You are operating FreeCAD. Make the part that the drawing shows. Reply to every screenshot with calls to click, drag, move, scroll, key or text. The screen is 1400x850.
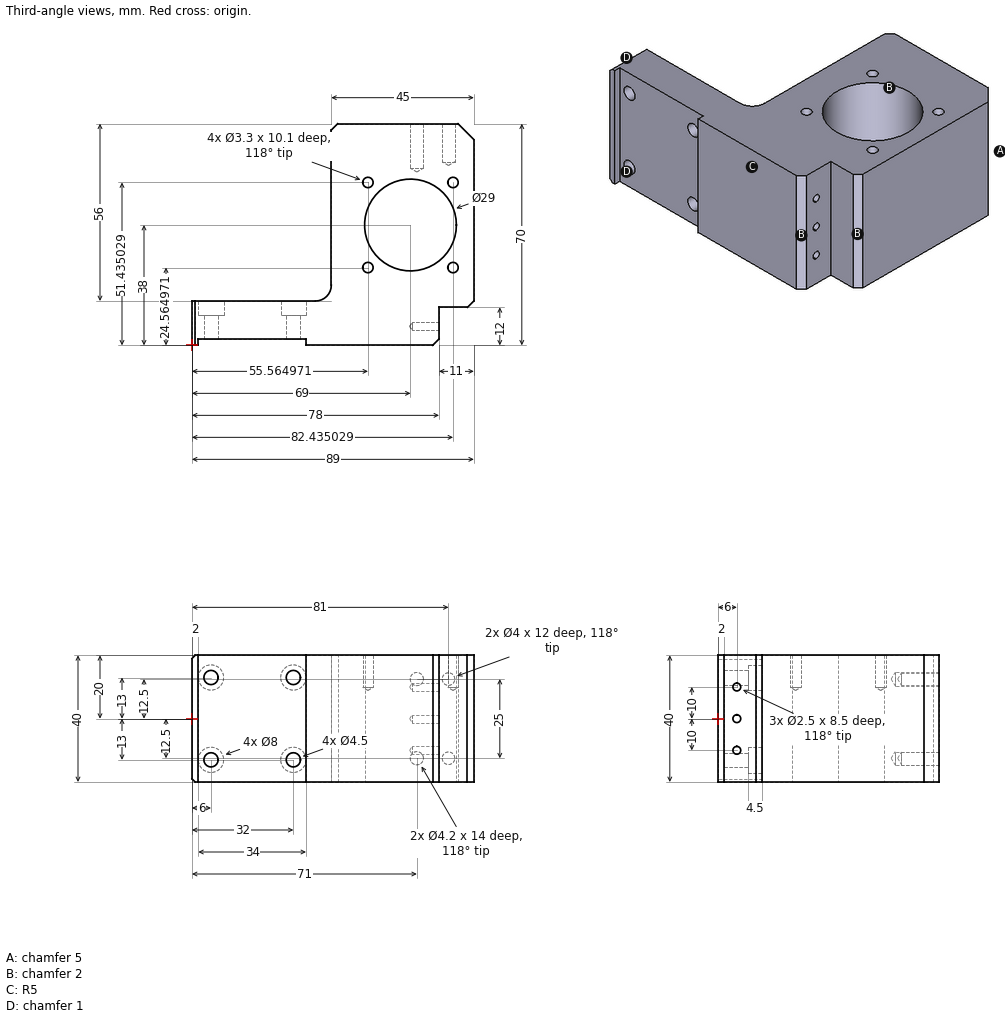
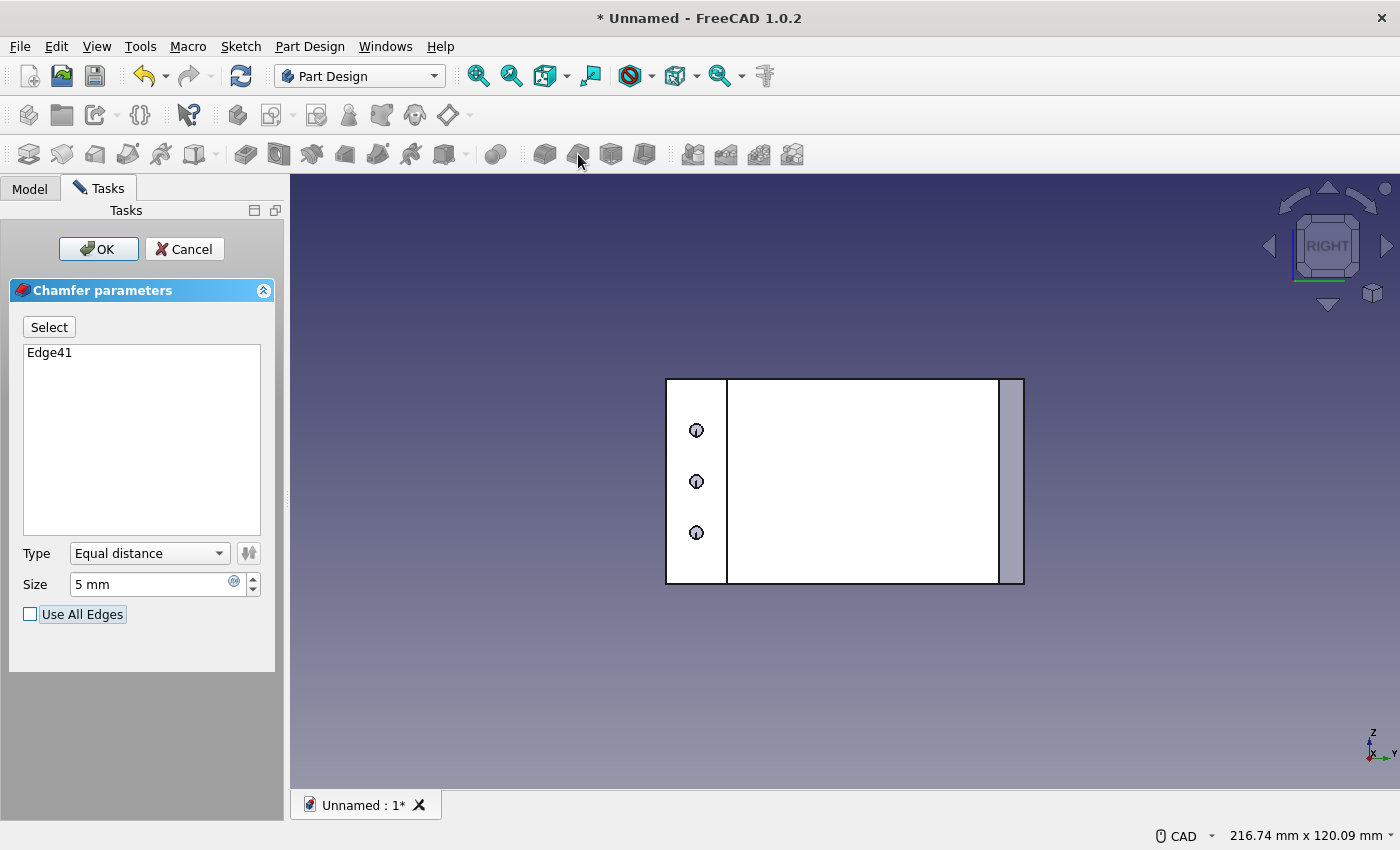
click(99, 249)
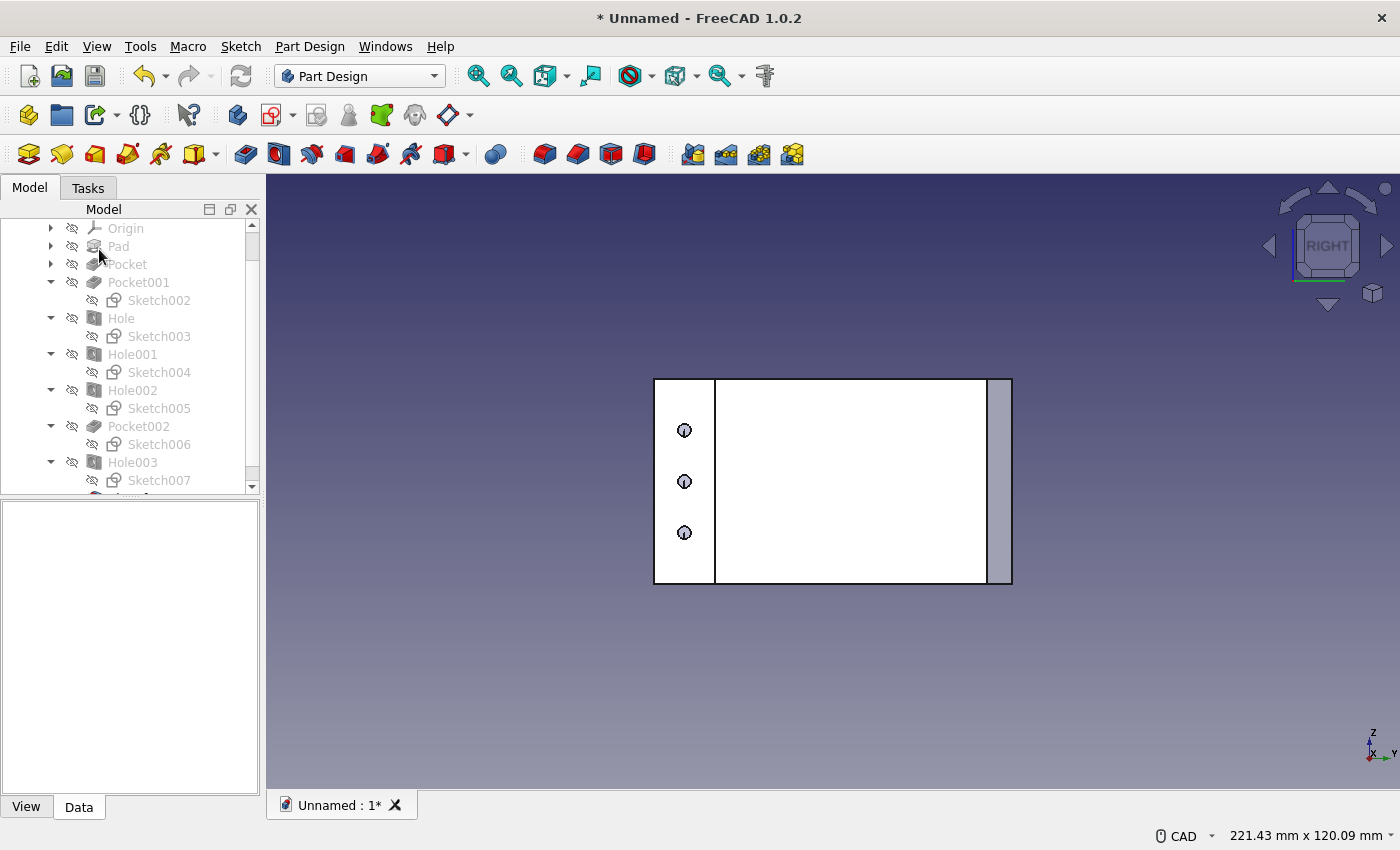
click(479, 76)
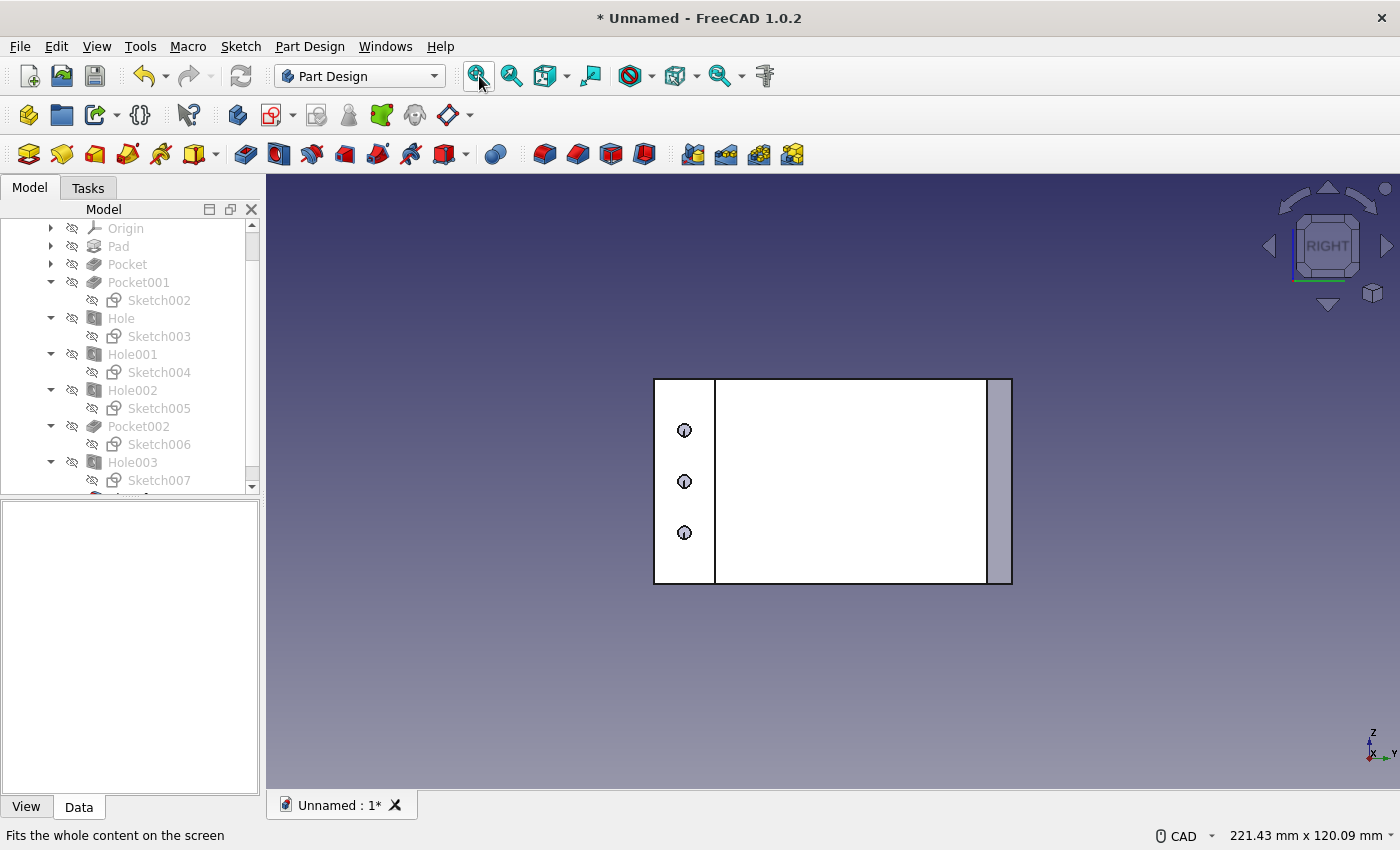
click(715, 480)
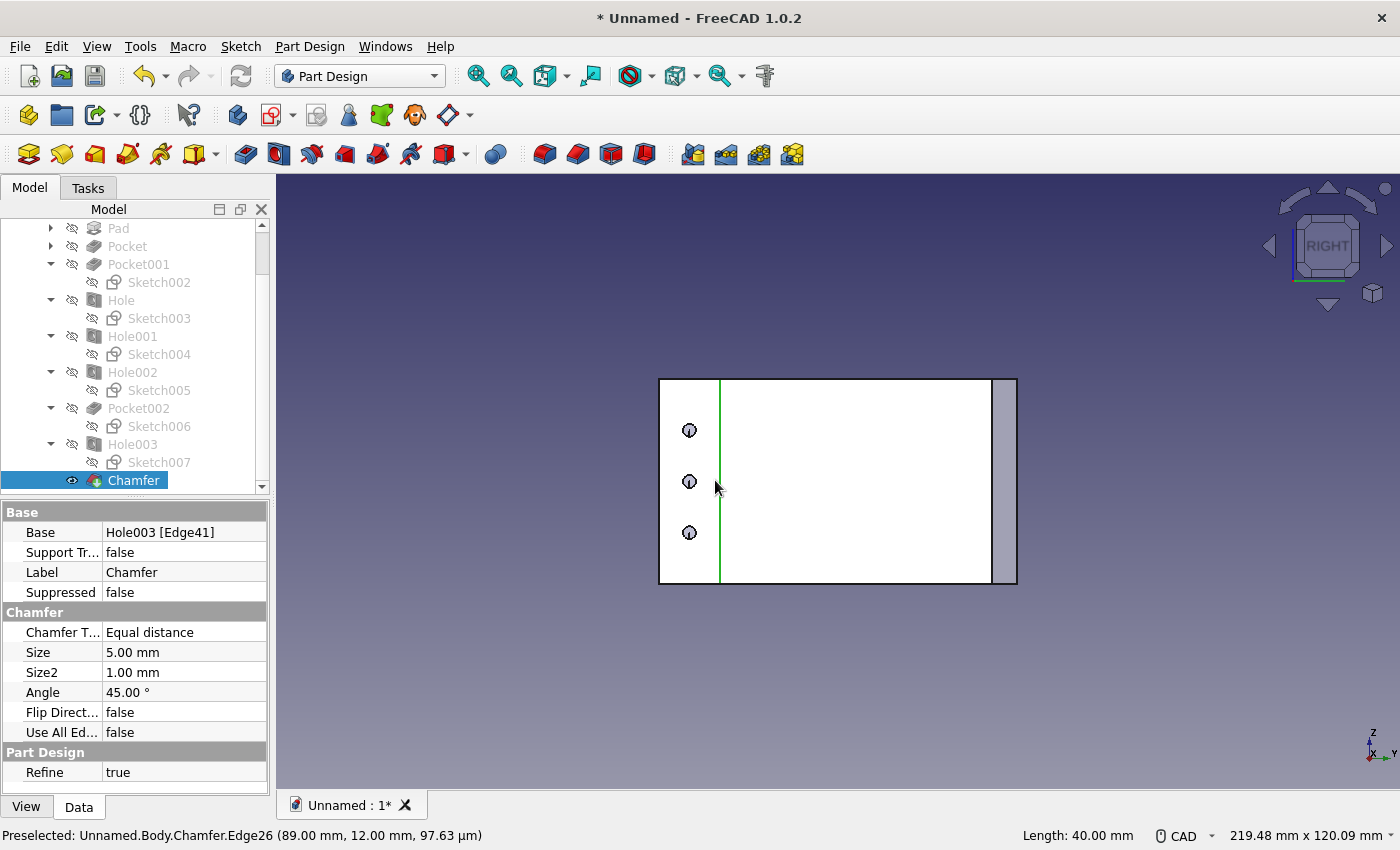
click(659, 480, ctrl)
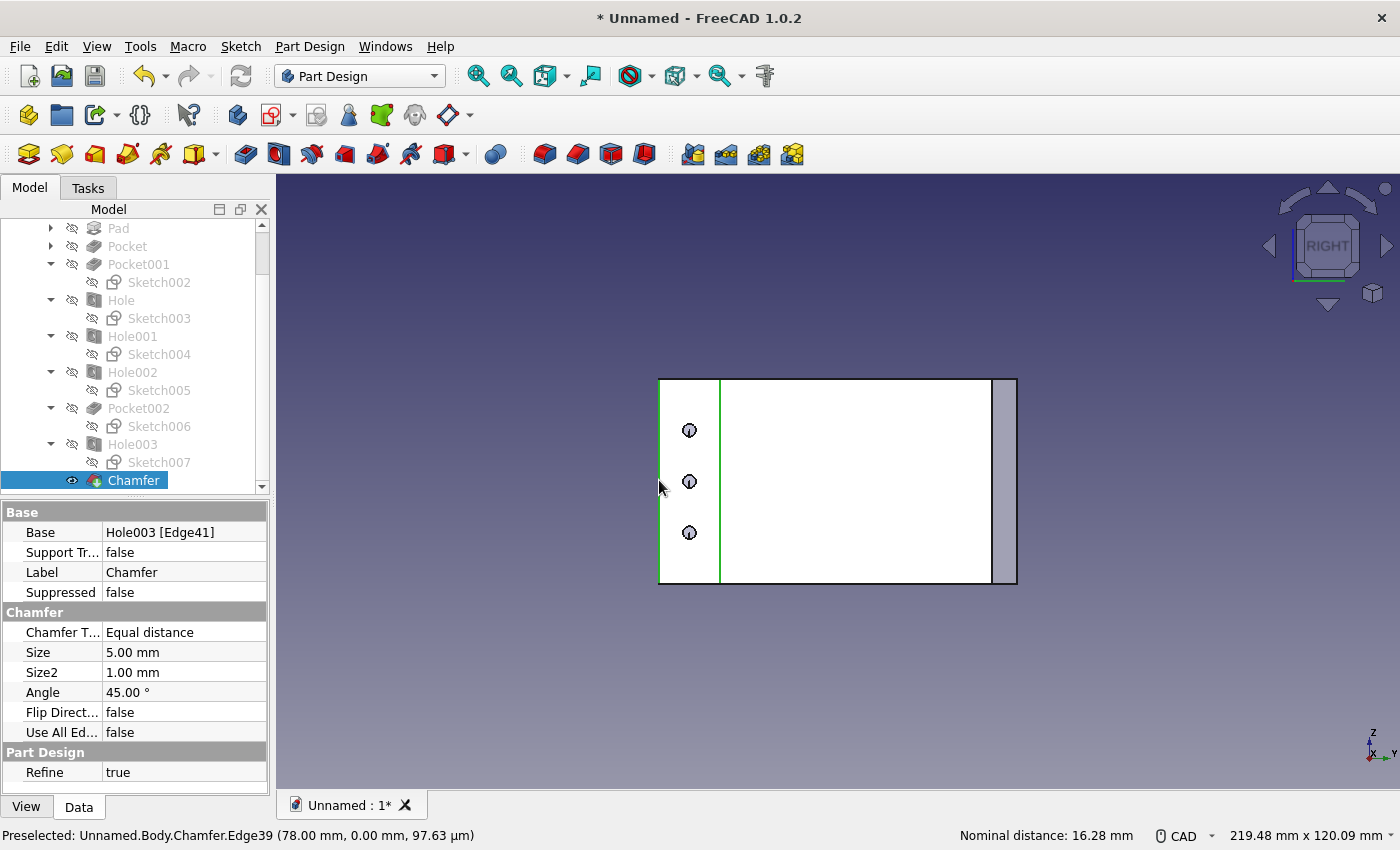
key(0)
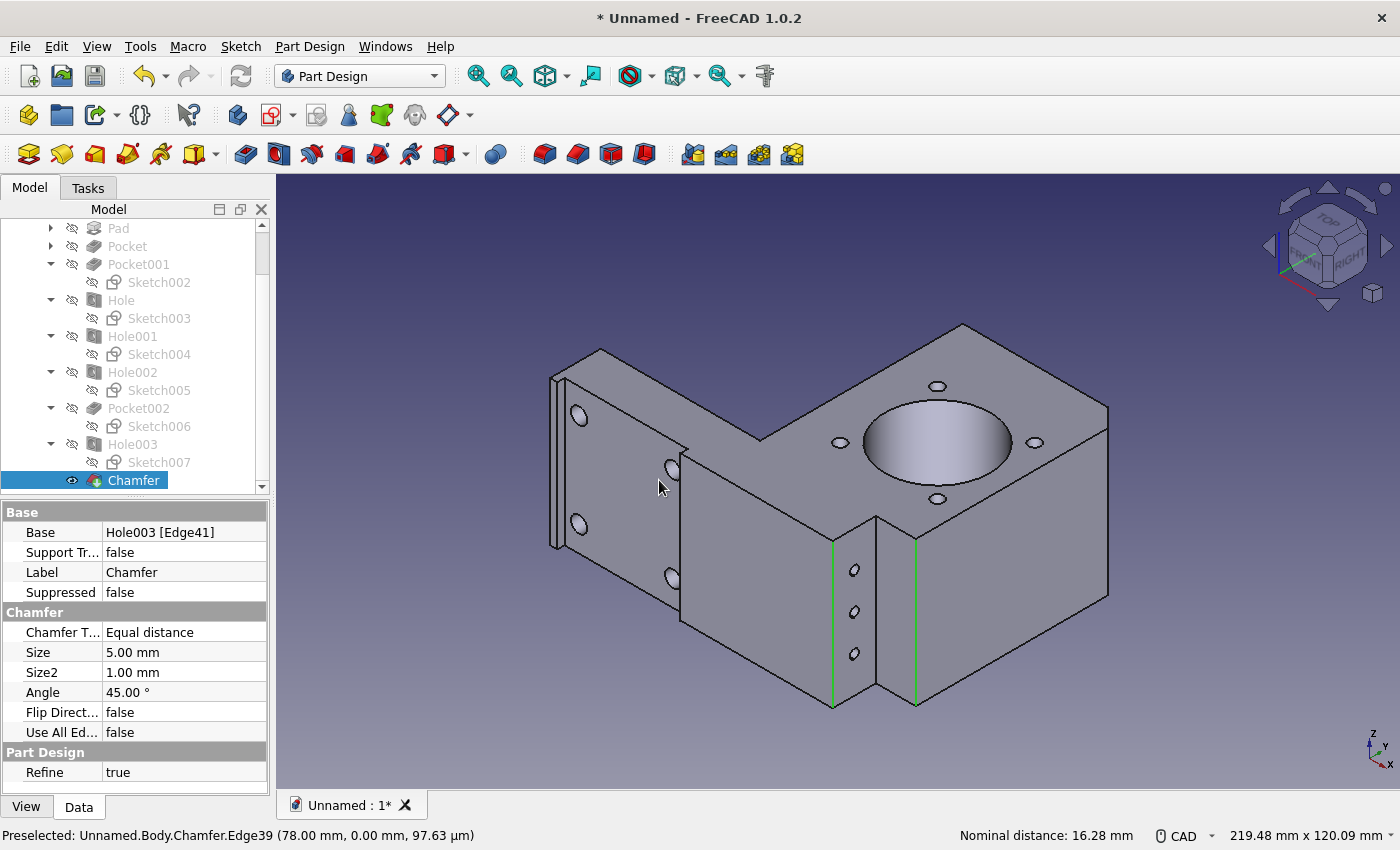
key(2)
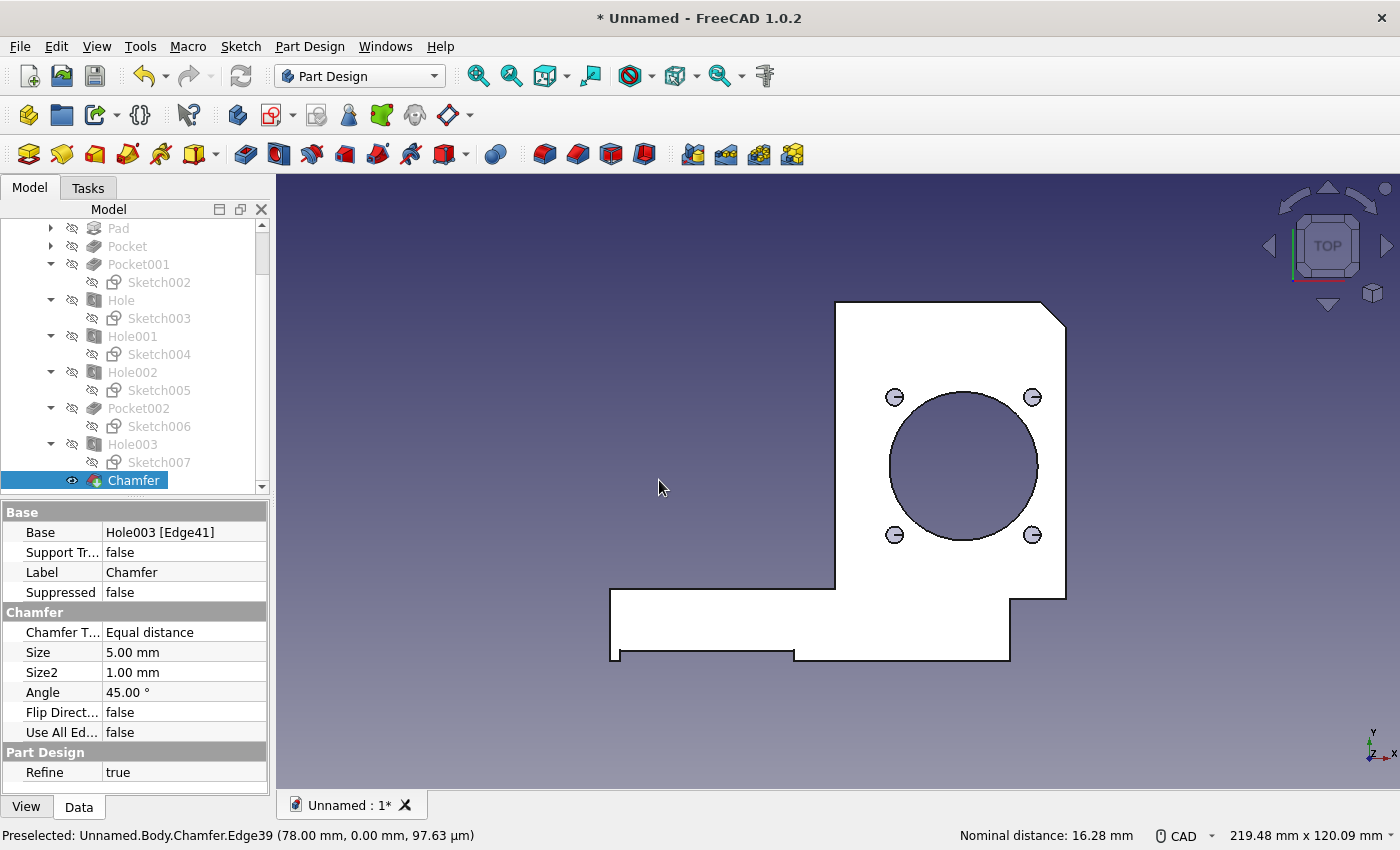
key(1)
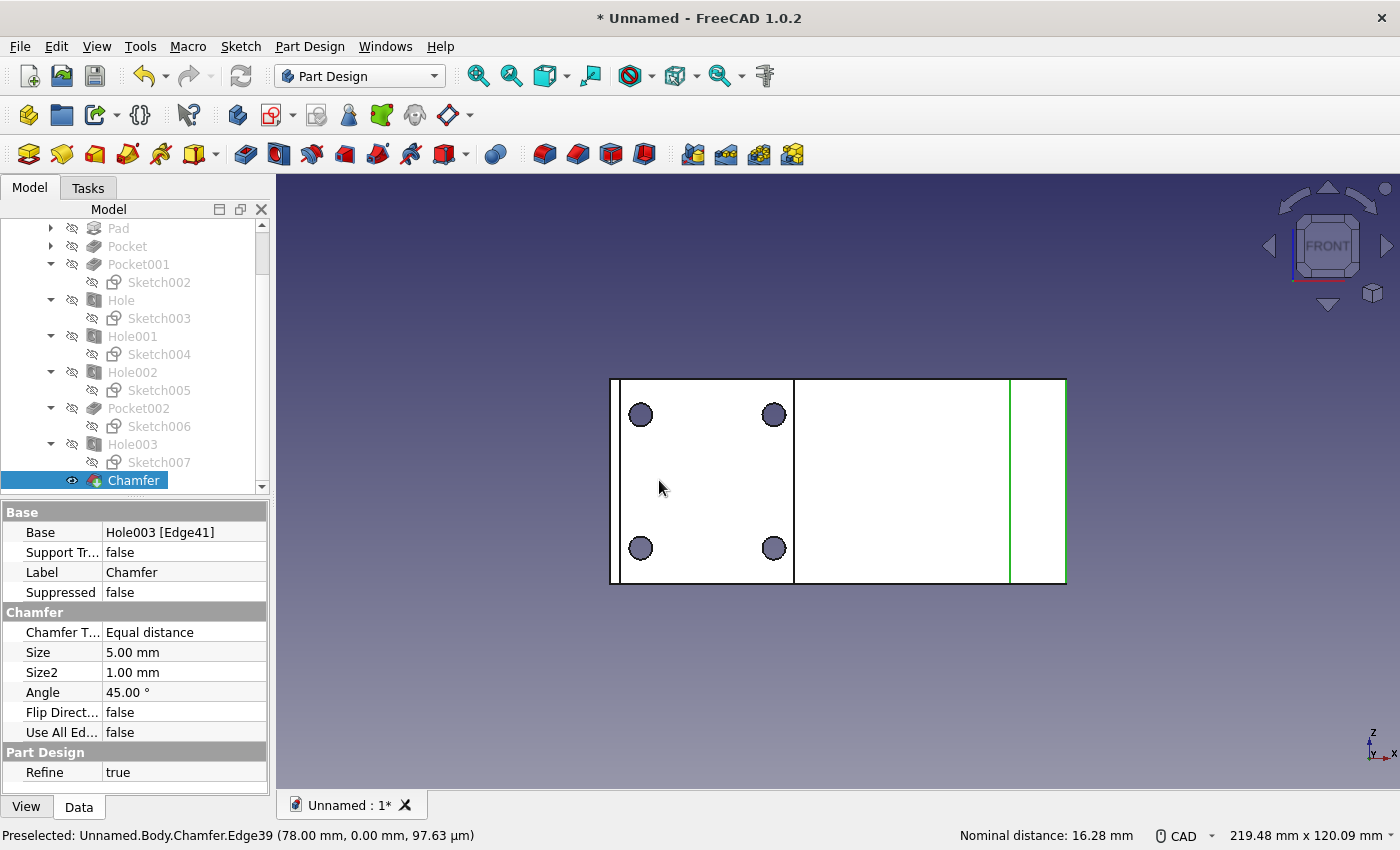
click(479, 76)